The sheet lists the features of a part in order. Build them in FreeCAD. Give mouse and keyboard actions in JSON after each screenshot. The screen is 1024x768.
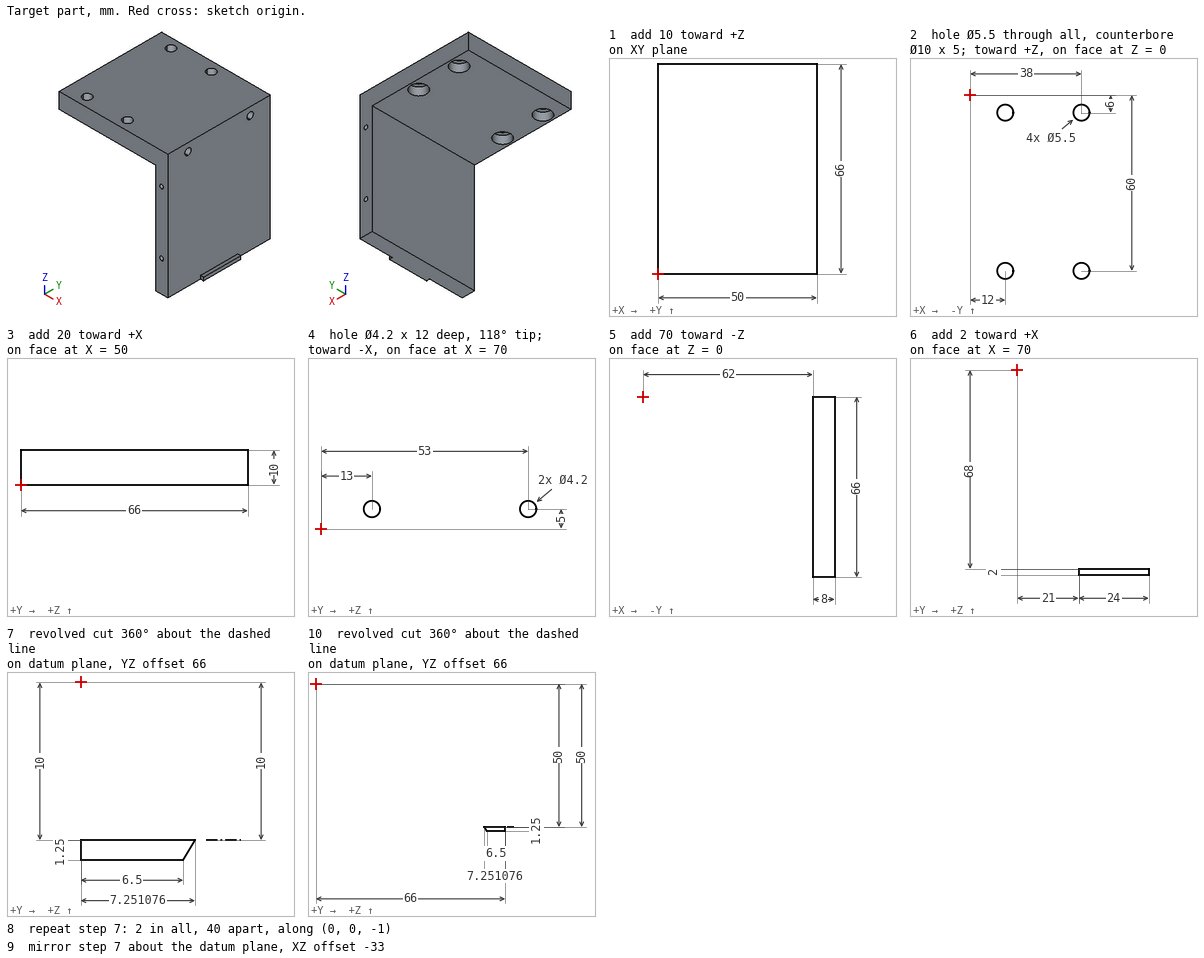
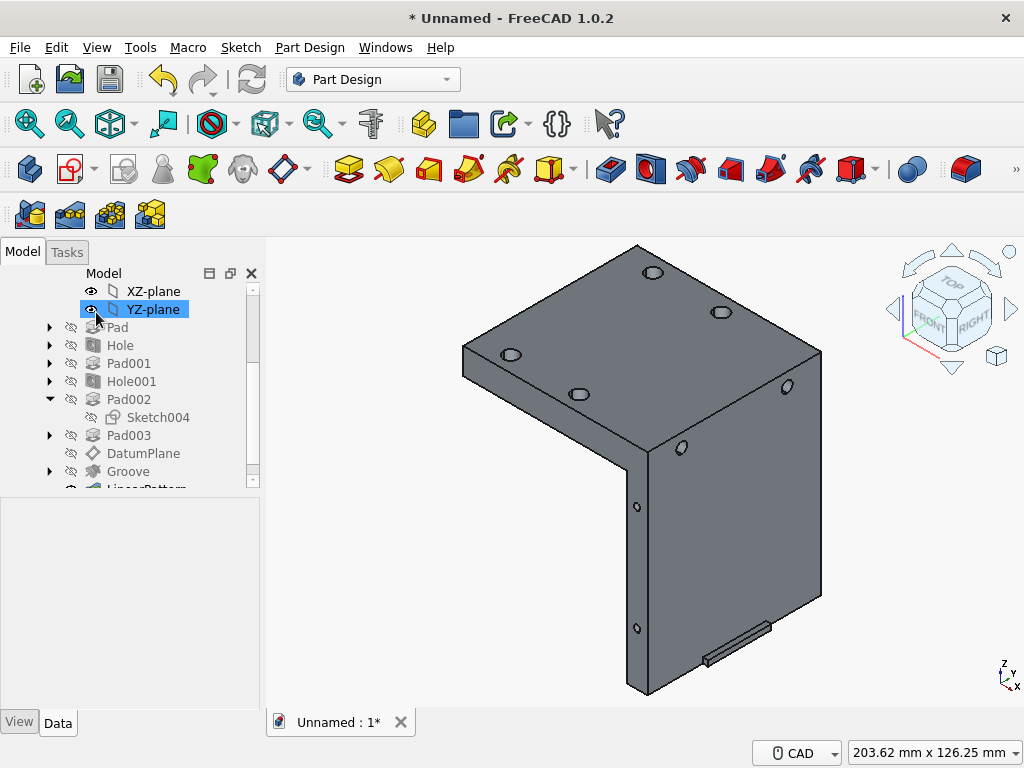
{"action": "scroll", "coordinate": [160, 377], "scroll_direction": "down", "scroll_amount": 3}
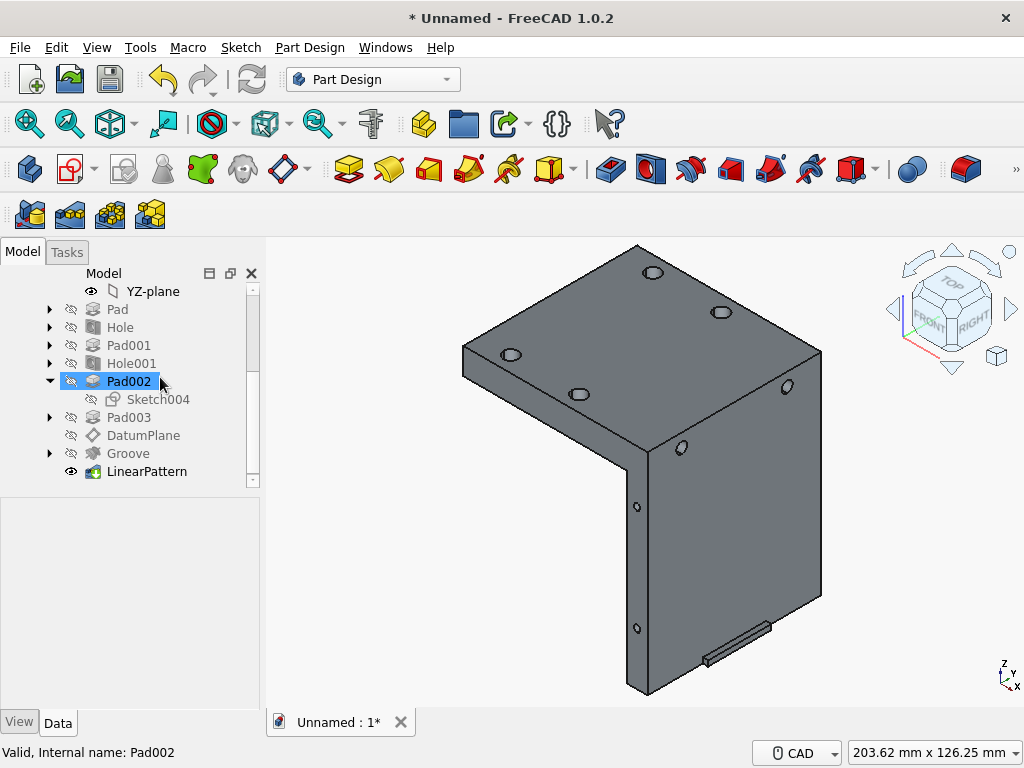
{"action": "scroll", "coordinate": [160, 377], "scroll_direction": "up", "scroll_amount": 15}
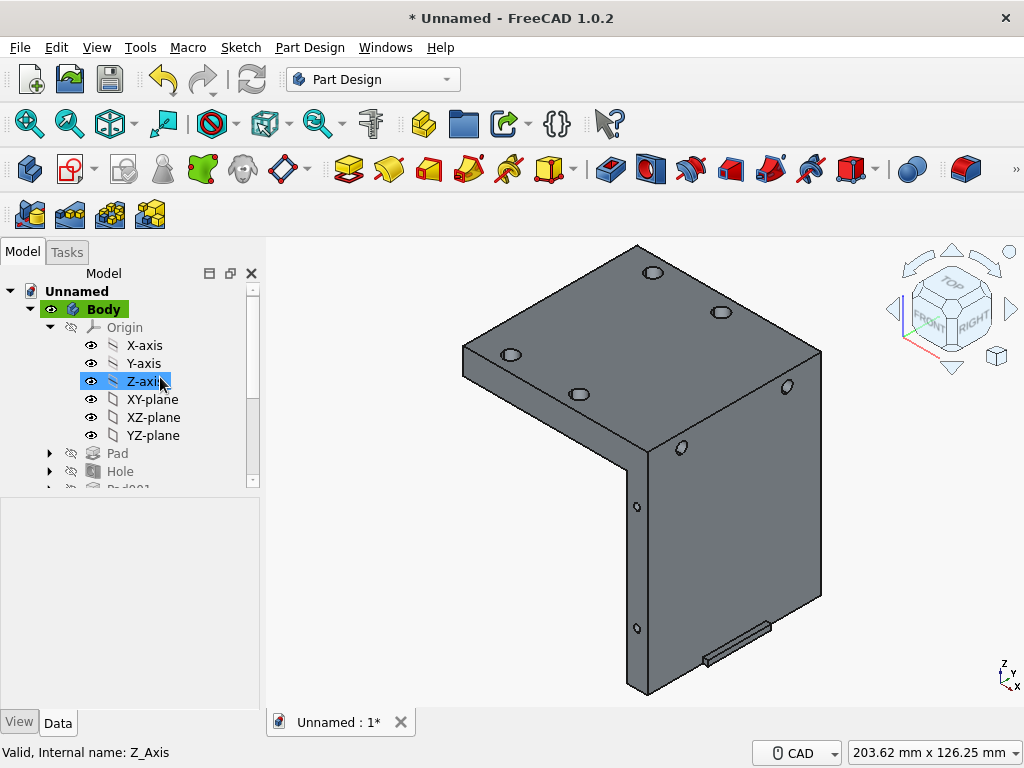
{"action": "left_click", "coordinate": [136, 417]}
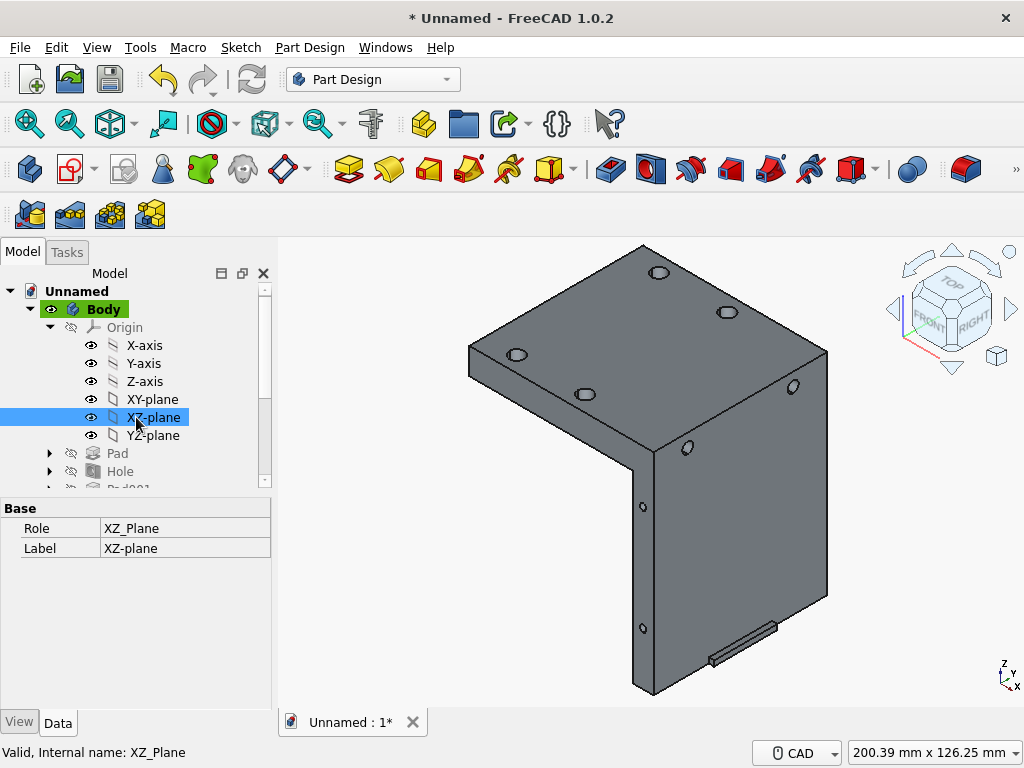
{"action": "left_click", "coordinate": [284, 170]}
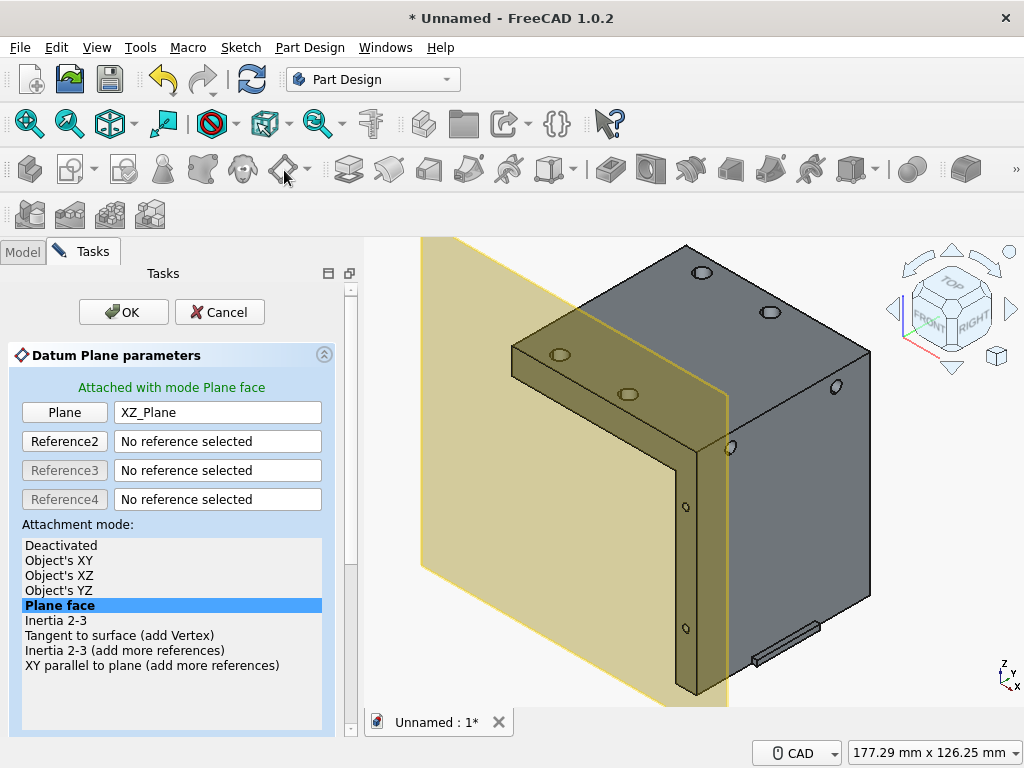
{"action": "scroll", "coordinate": [351, 510], "scroll_direction": "down", "scroll_amount": 3}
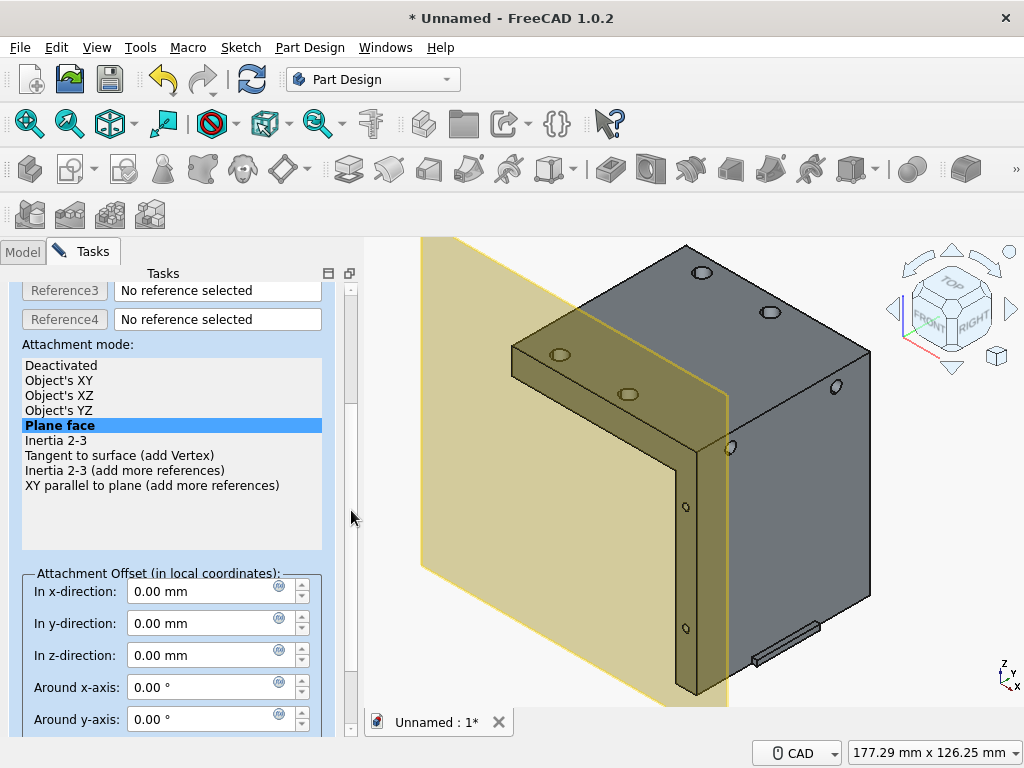
{"action": "triple_click", "coordinate": [210, 655]}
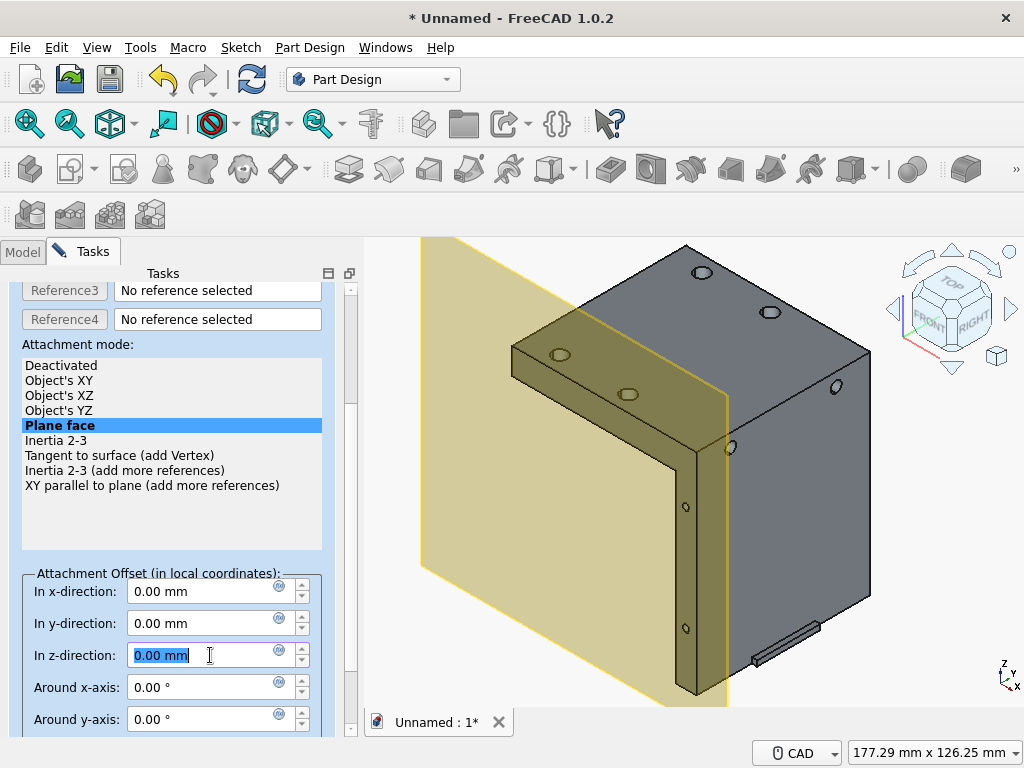
{"action": "type", "text": "-33"}
{"action": "key", "text": "Tab"}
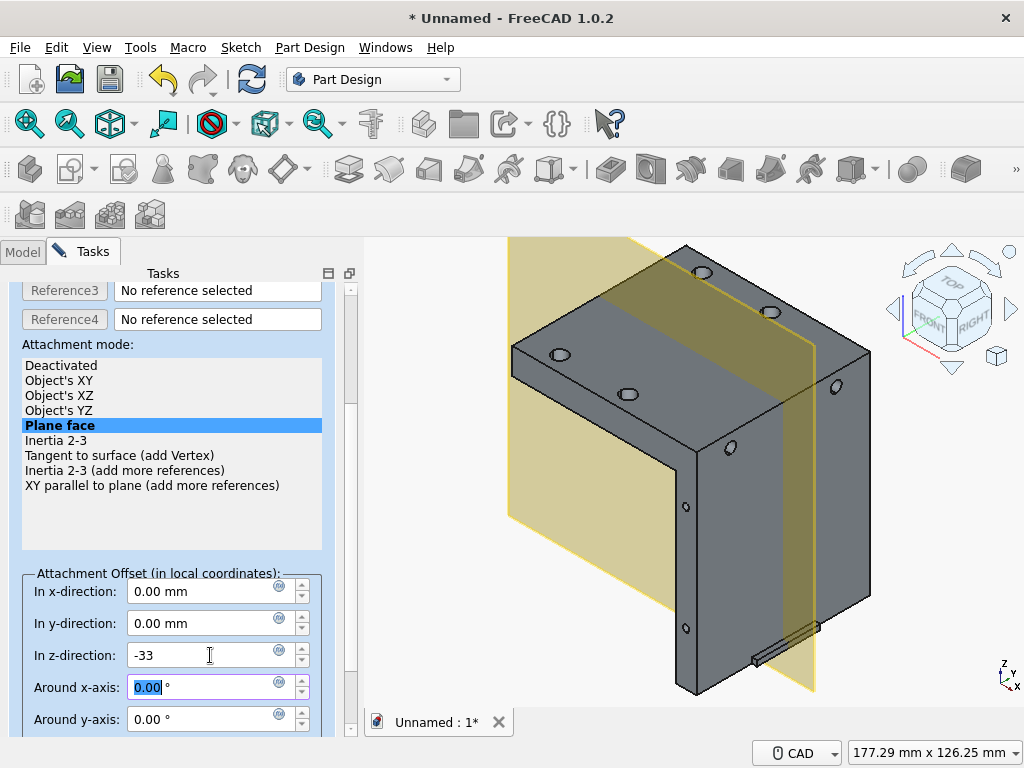
{"action": "scroll", "coordinate": [351, 510], "scroll_direction": "up", "scroll_amount": 4}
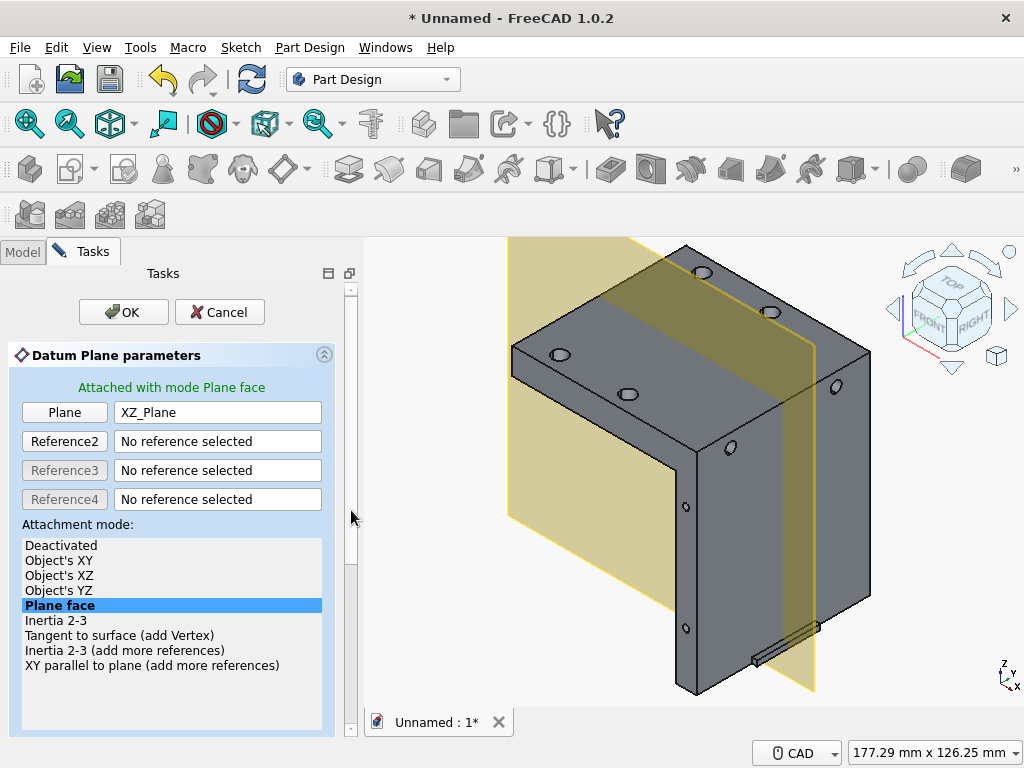
{"action": "left_click", "coordinate": [124, 312]}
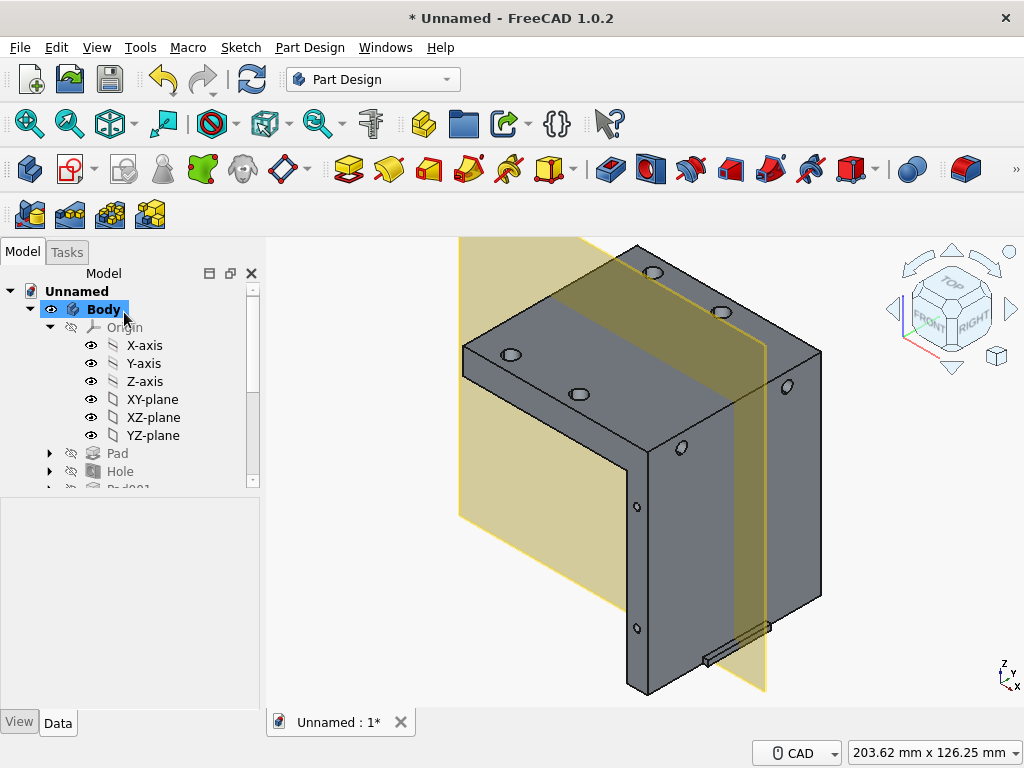
{"action": "scroll", "coordinate": [100, 377], "scroll_direction": "down", "scroll_amount": 3}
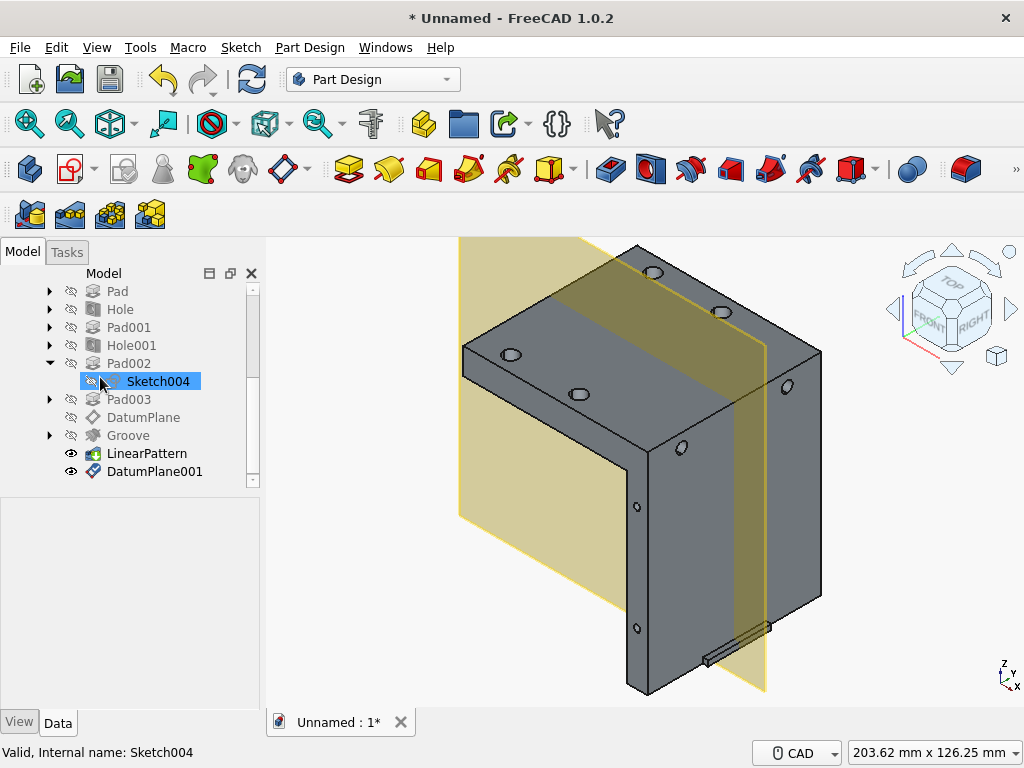
{"action": "left_click", "coordinate": [116, 435]}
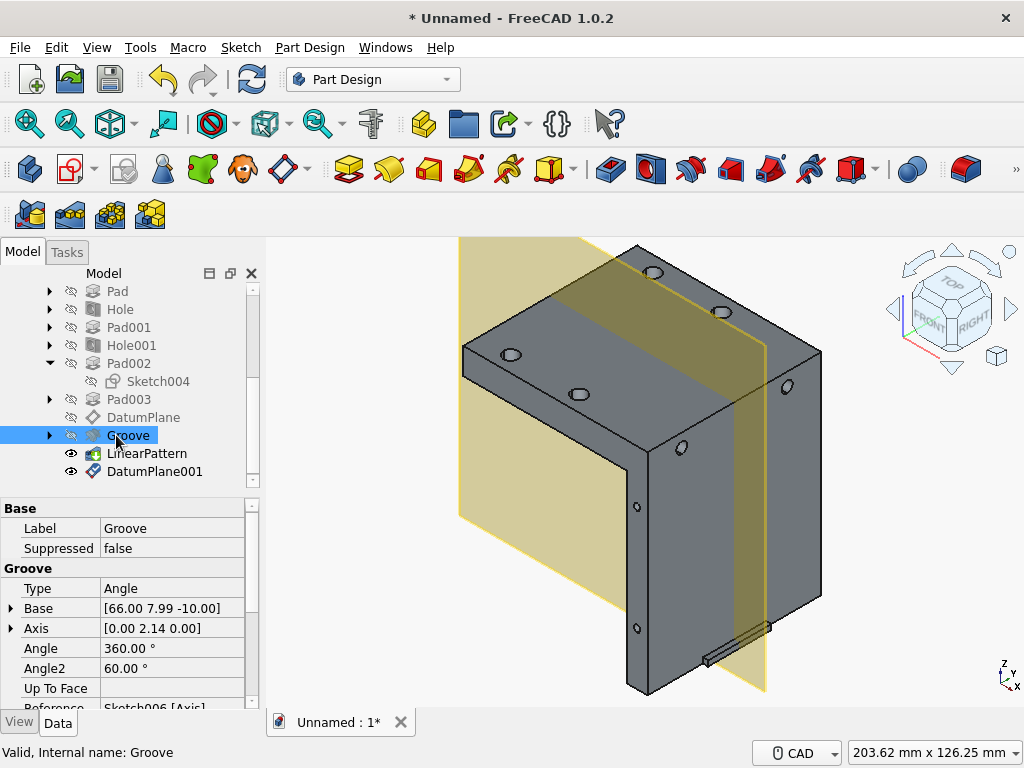
{"action": "left_click", "coordinate": [30, 214]}